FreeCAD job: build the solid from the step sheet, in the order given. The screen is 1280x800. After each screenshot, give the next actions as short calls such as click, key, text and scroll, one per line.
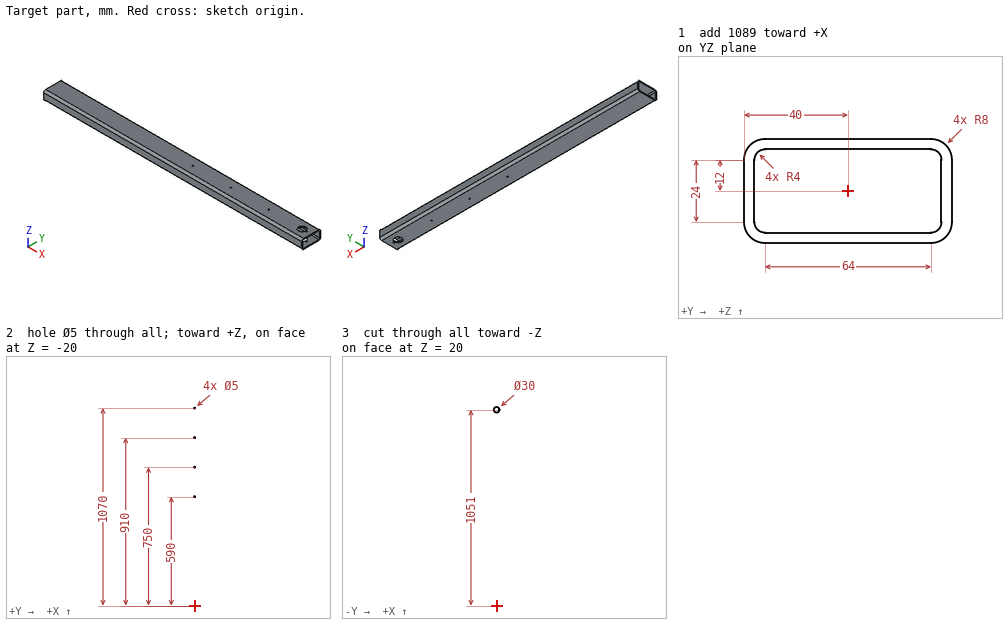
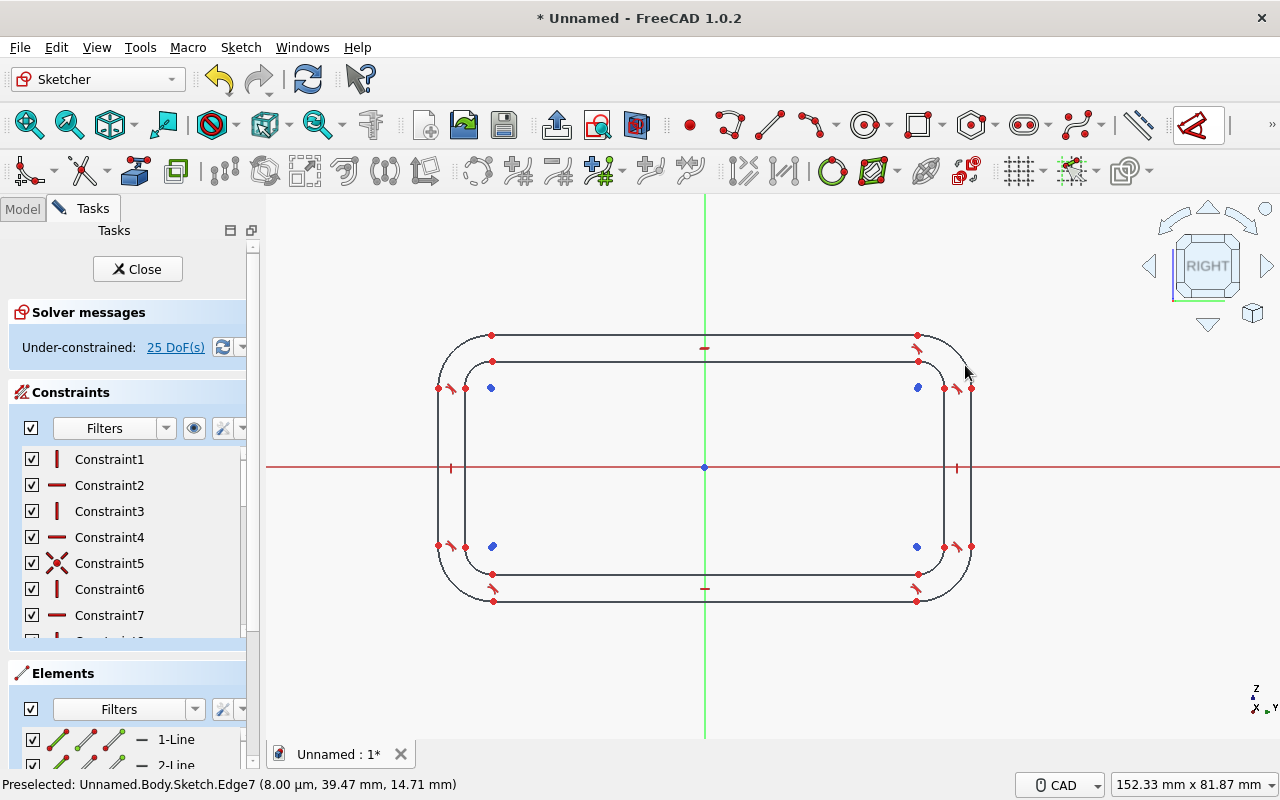
click(790, 335)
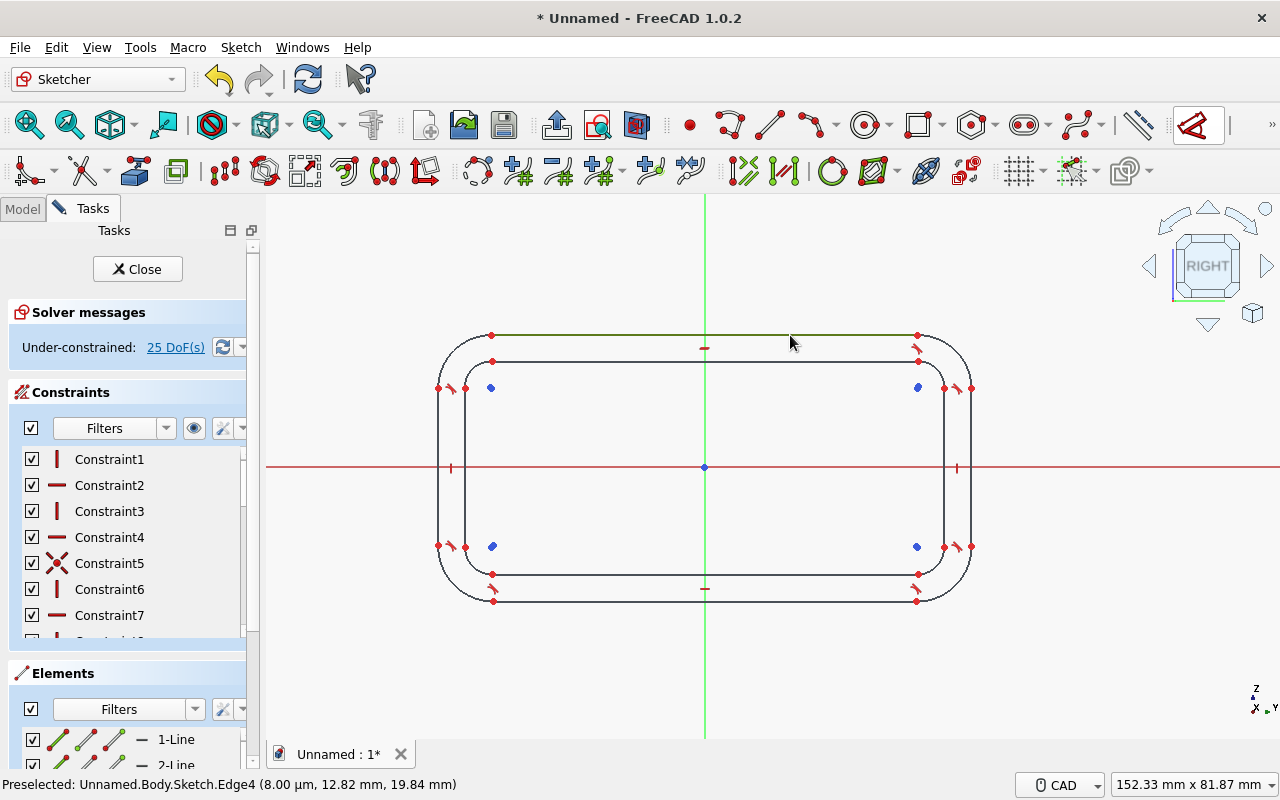
click(467, 341)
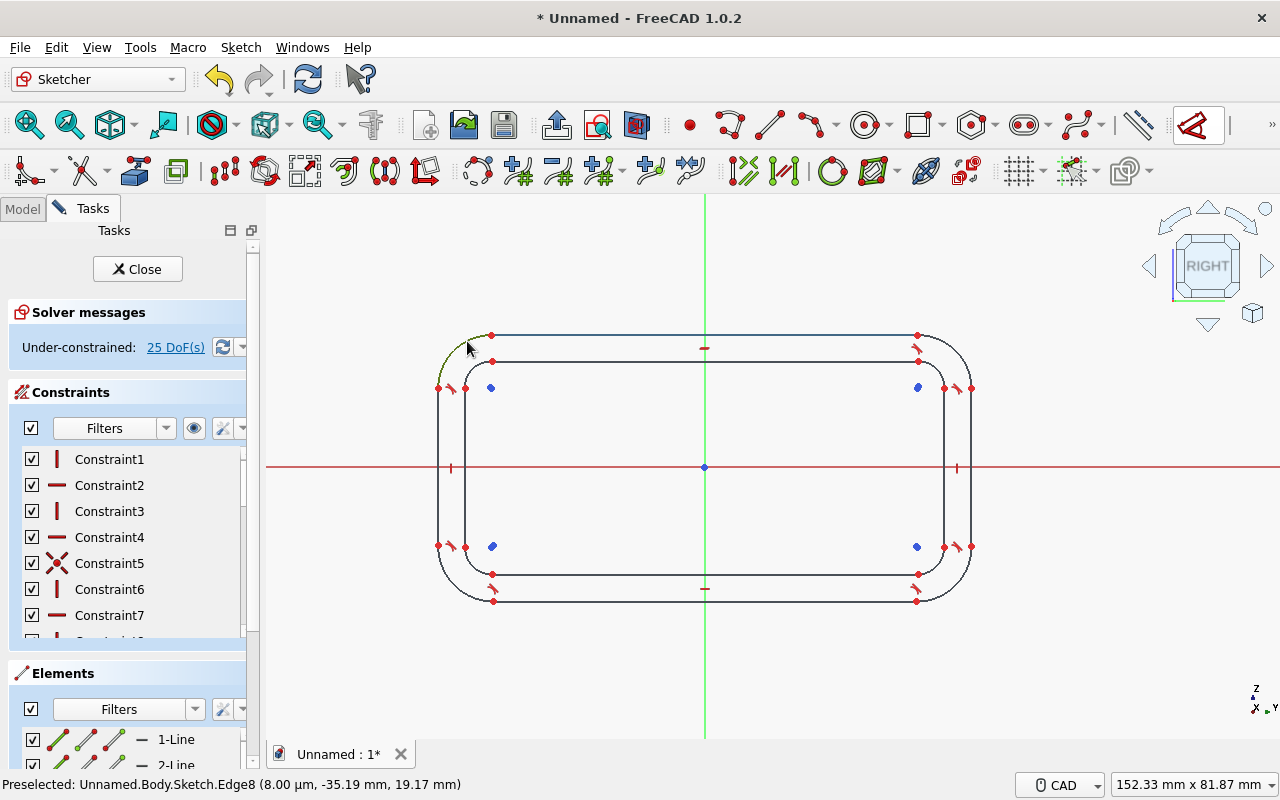
key(t)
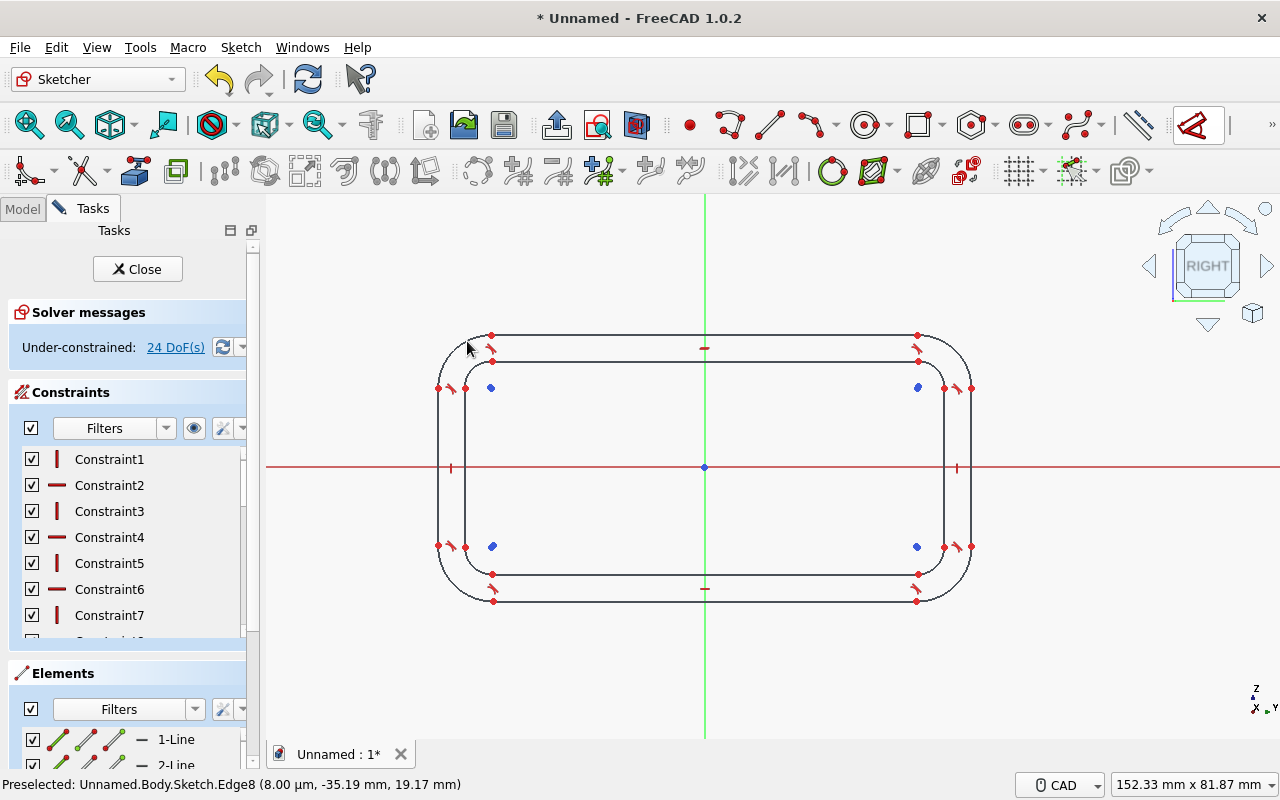
click(465, 500)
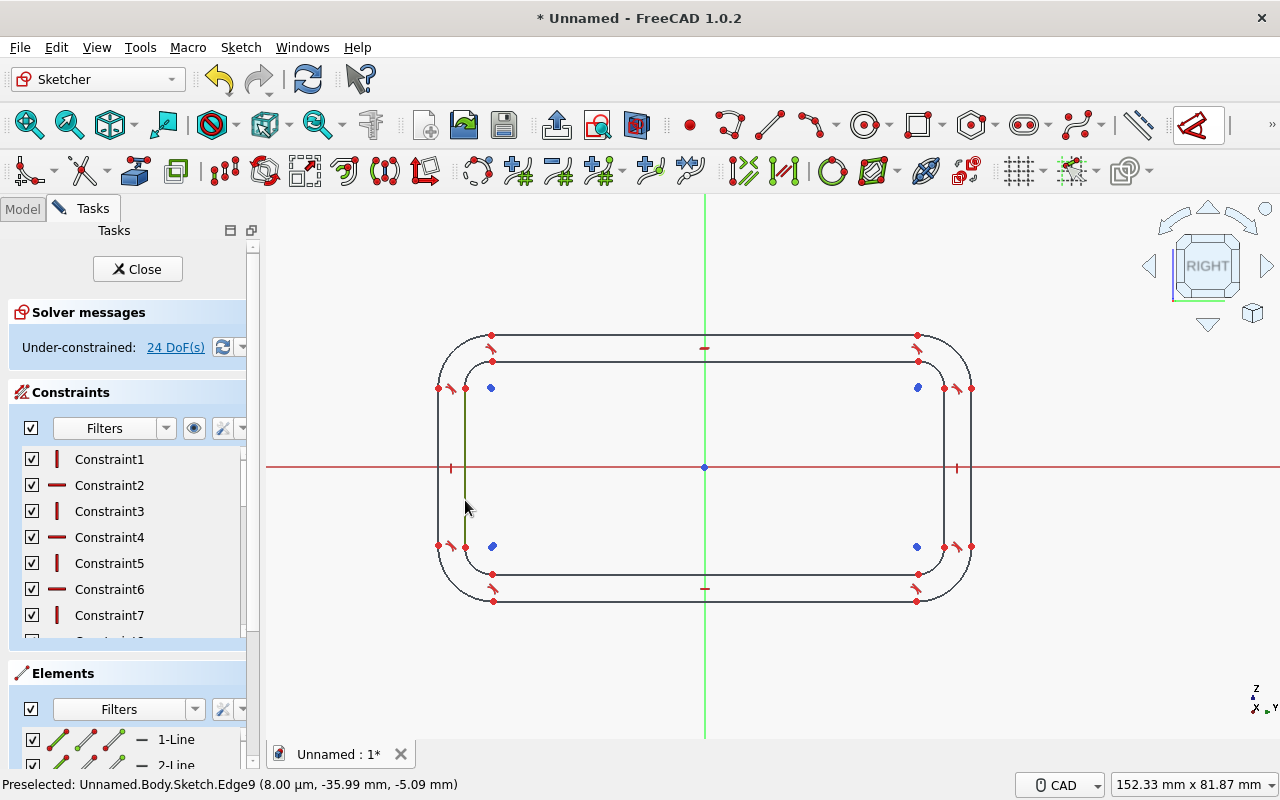
click(479, 364)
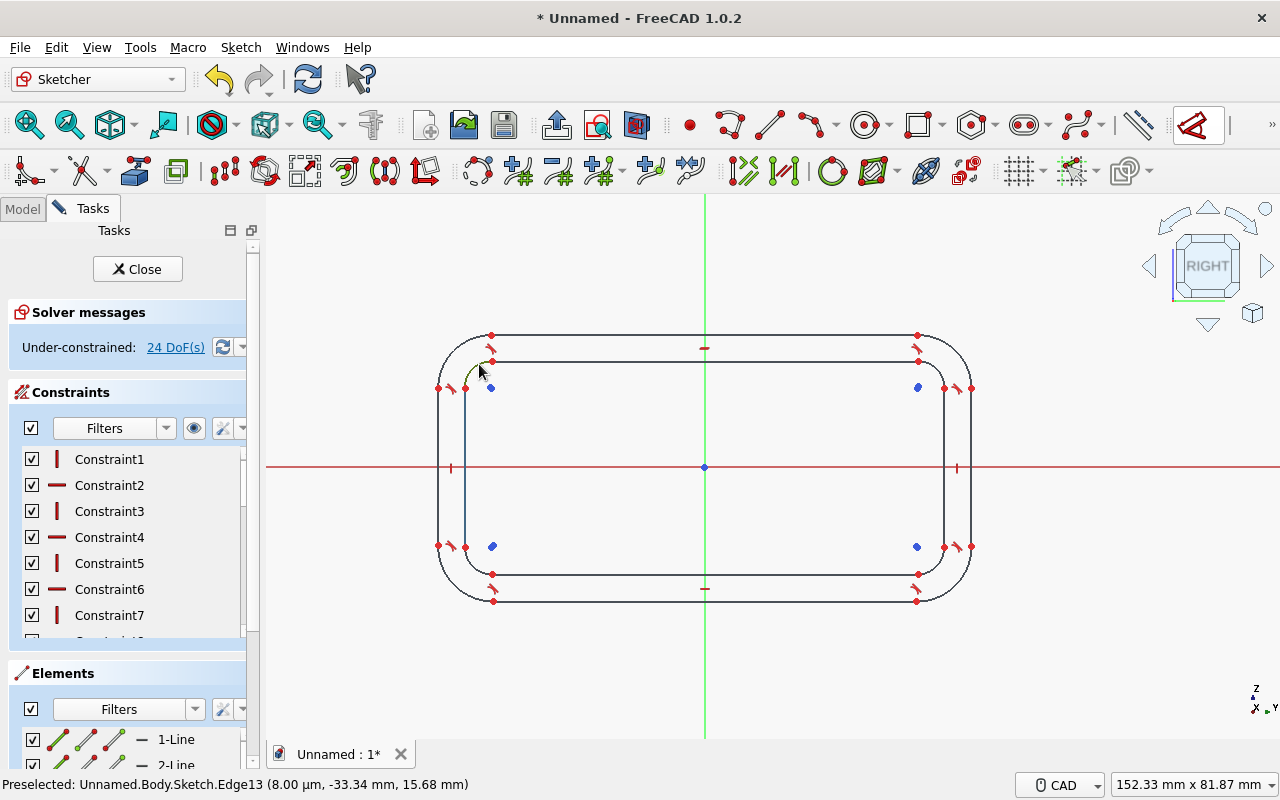
key(t)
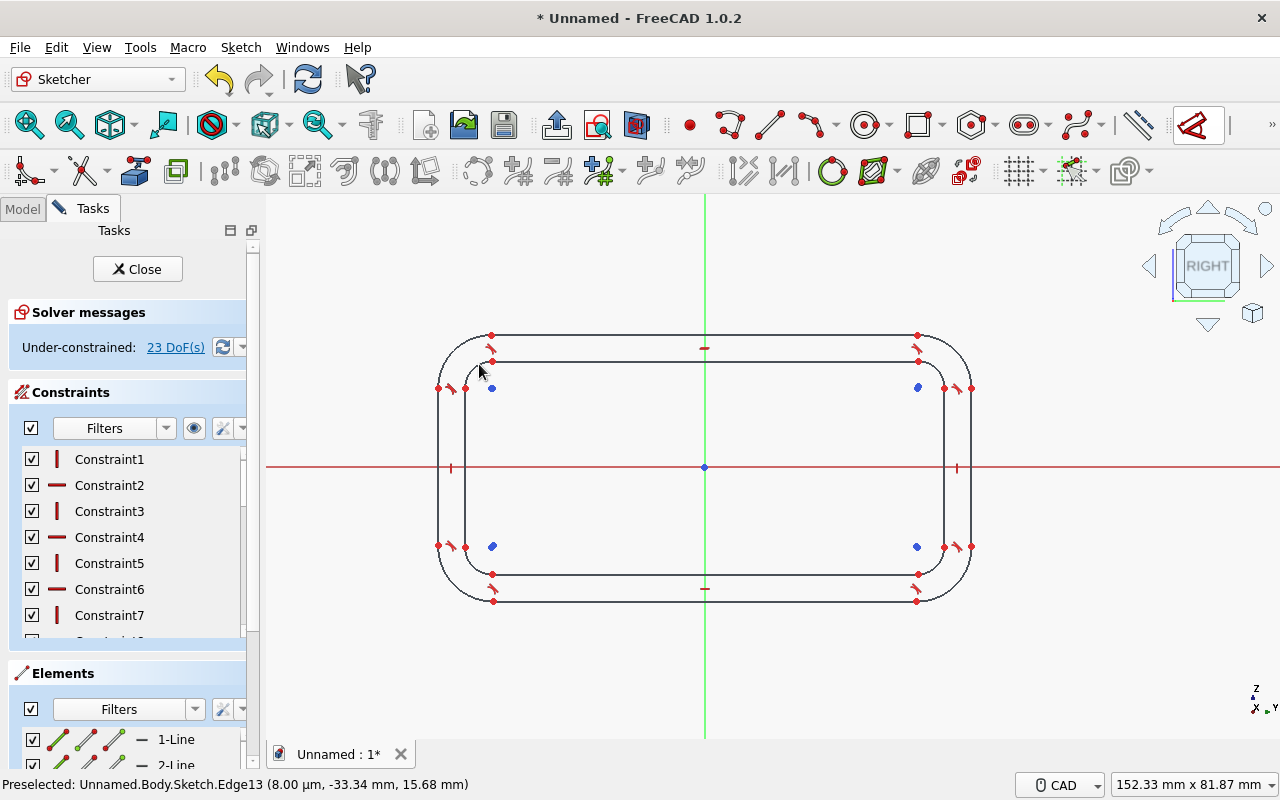
click(465, 500)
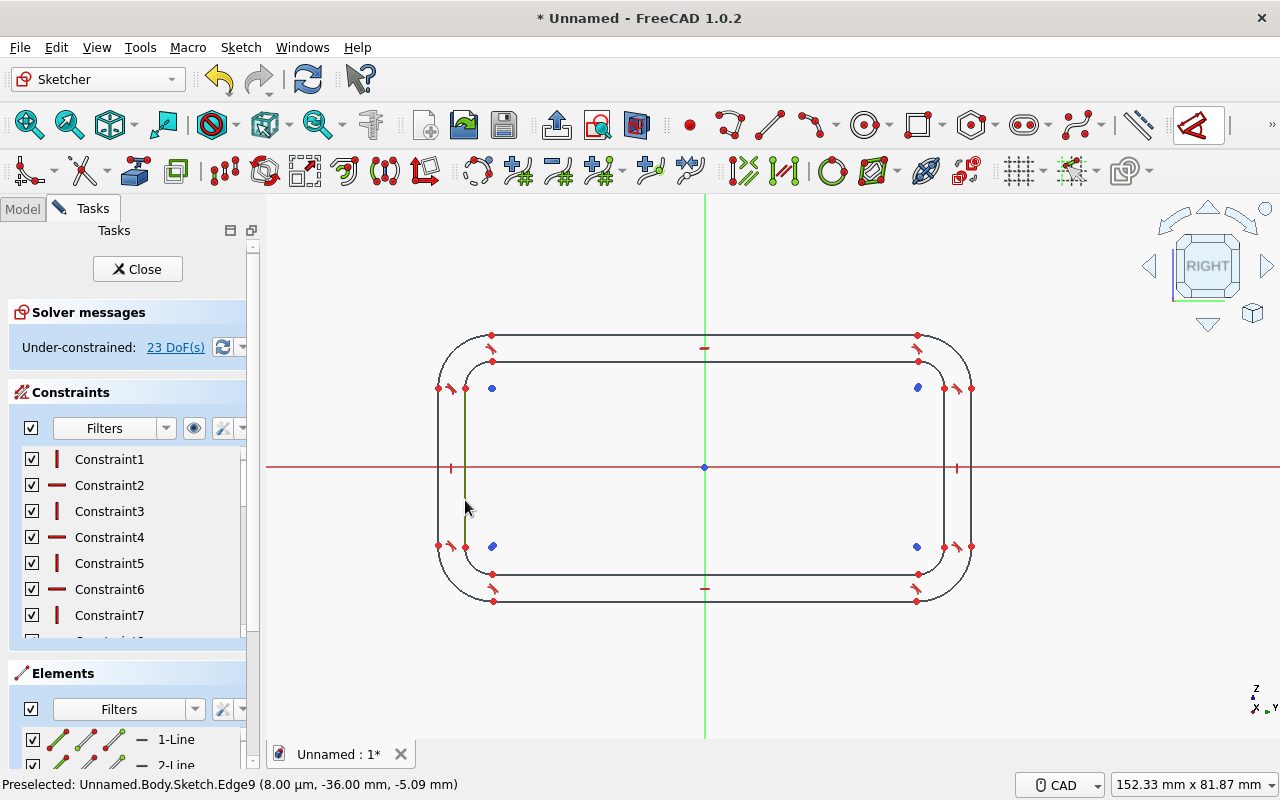
click(468, 560)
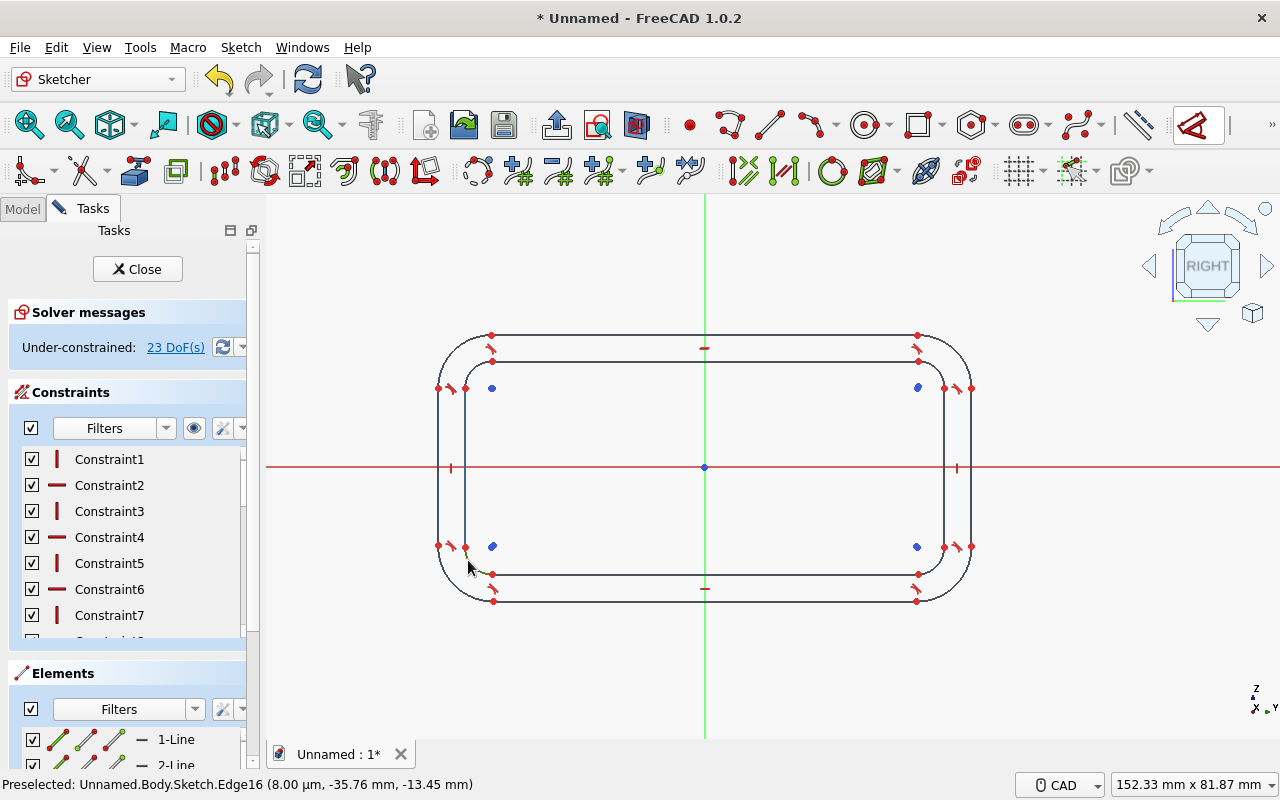
key(t)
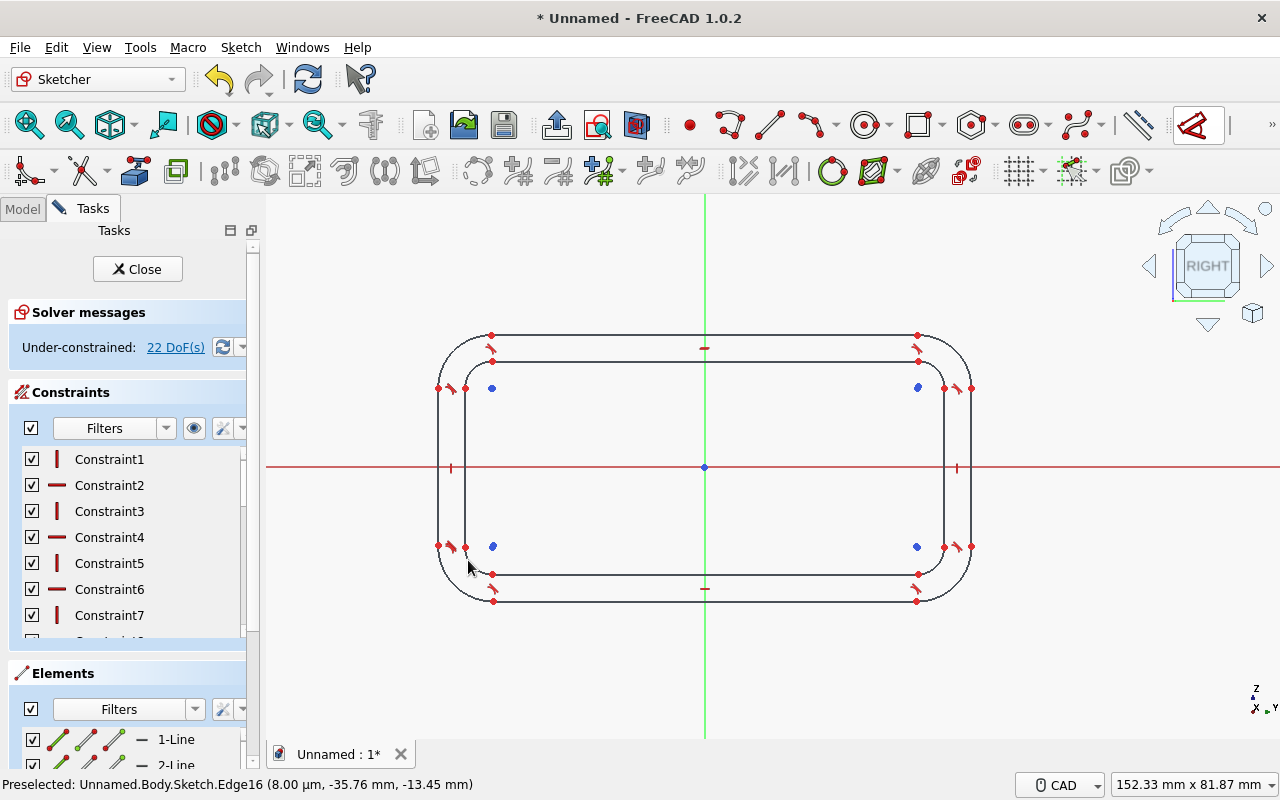
click(620, 362)